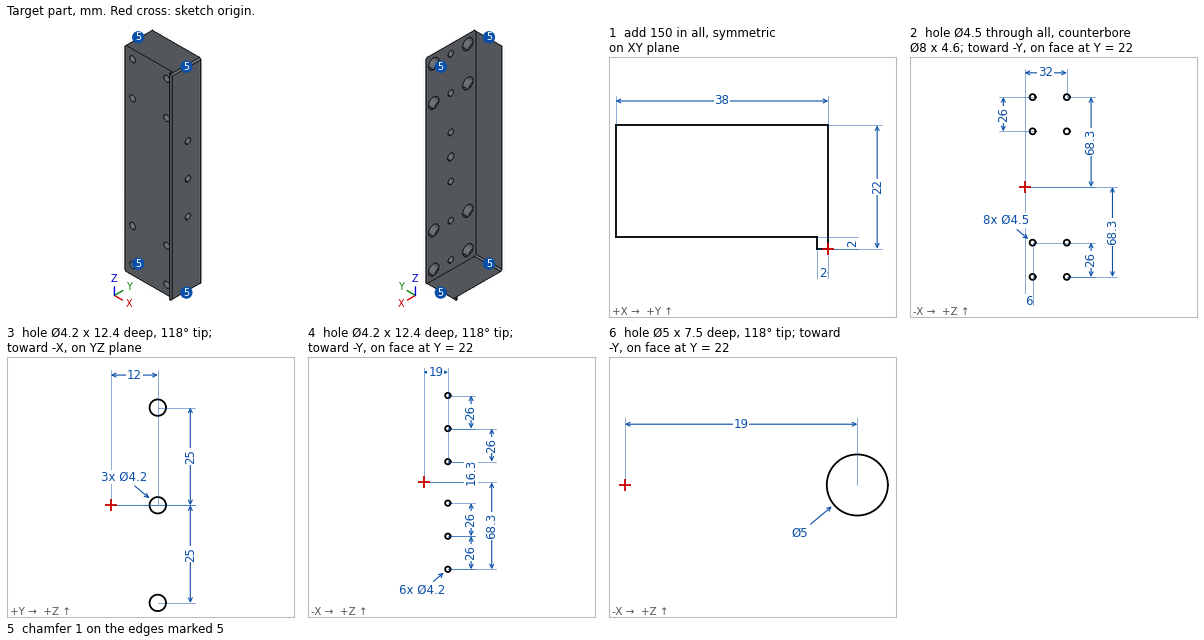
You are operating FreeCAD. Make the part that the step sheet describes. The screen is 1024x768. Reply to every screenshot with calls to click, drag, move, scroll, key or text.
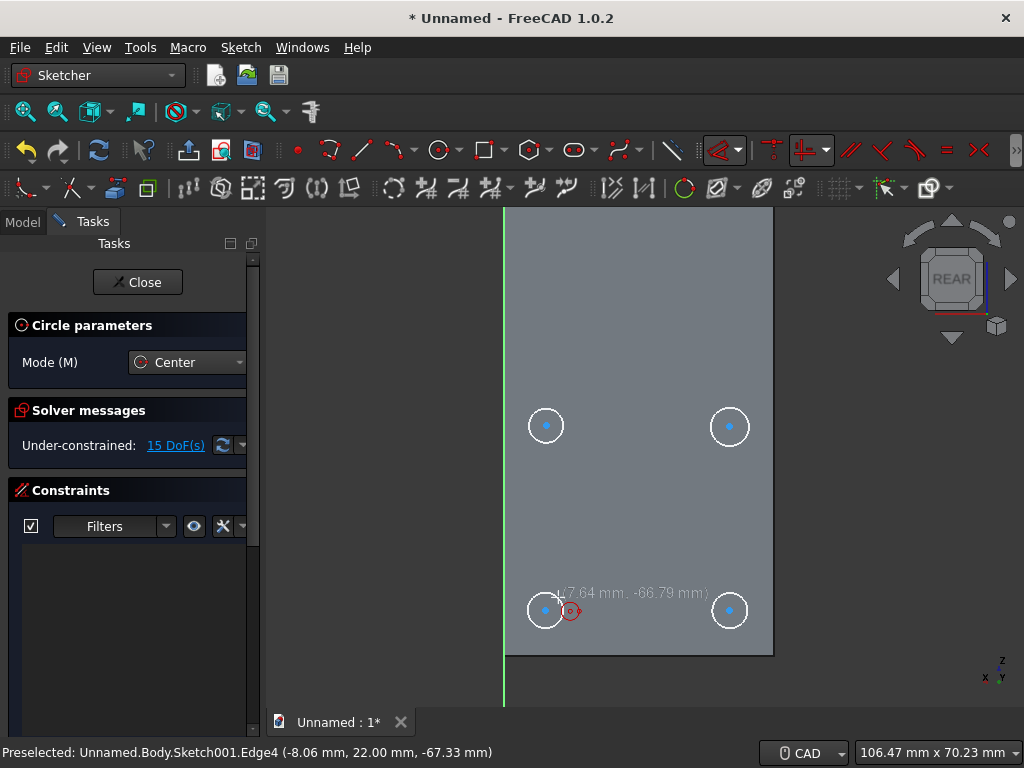
scroll(555, 601, down, 6)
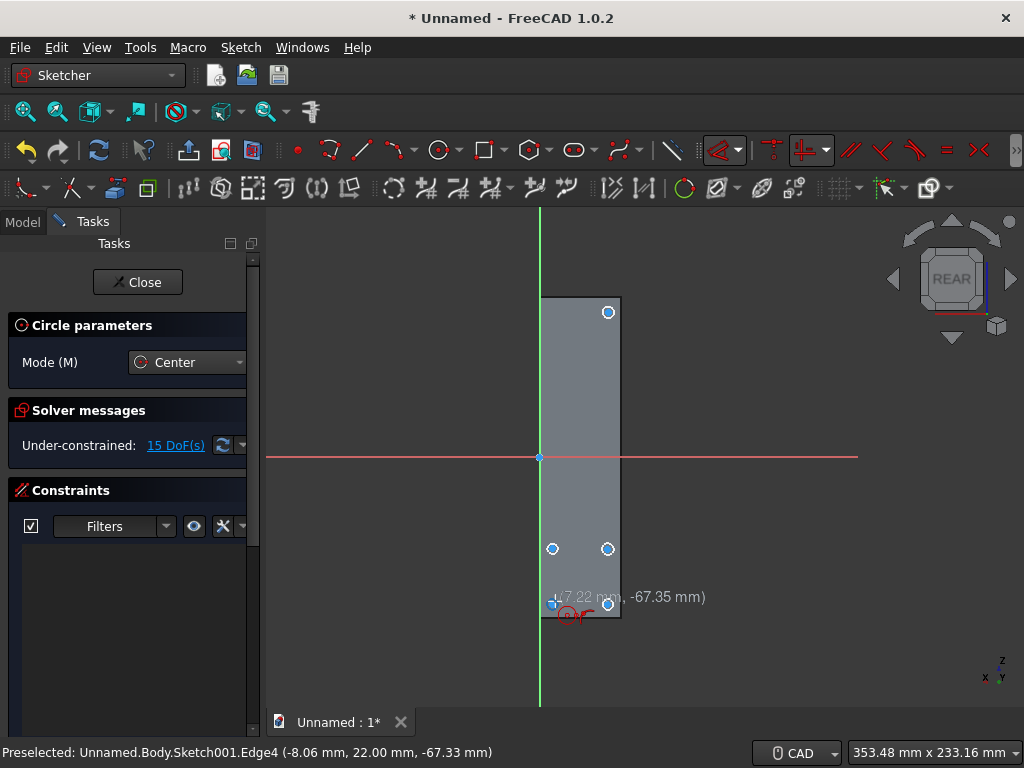
scroll(553, 311, up, 8)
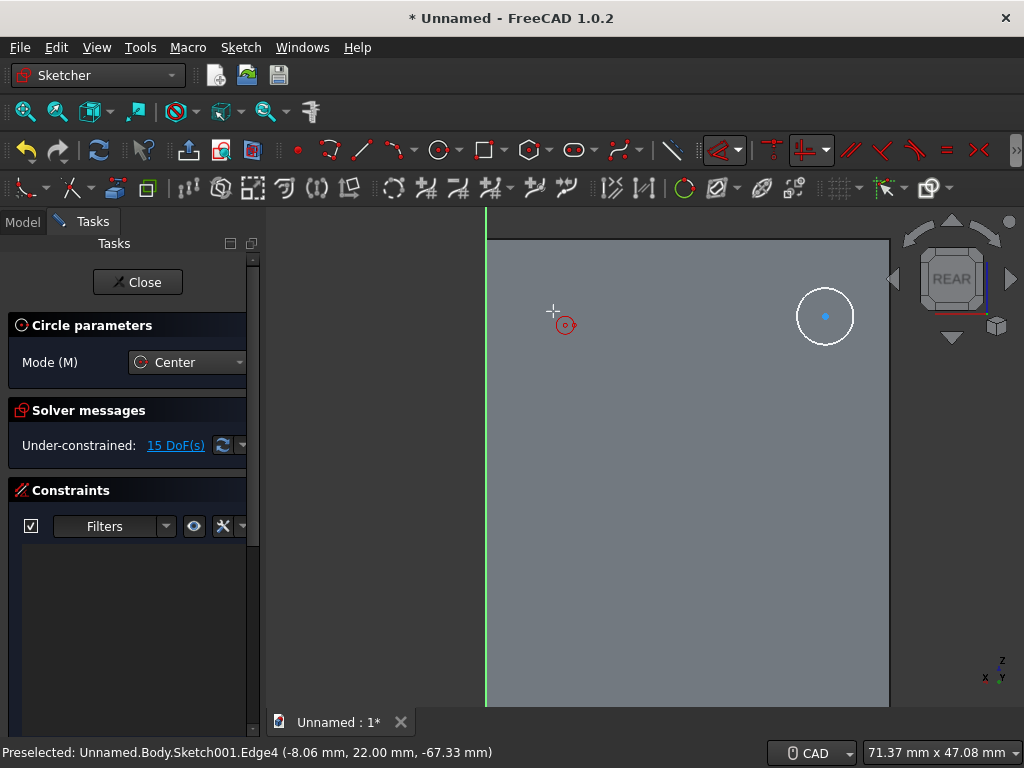
scroll(553, 311, down, 8)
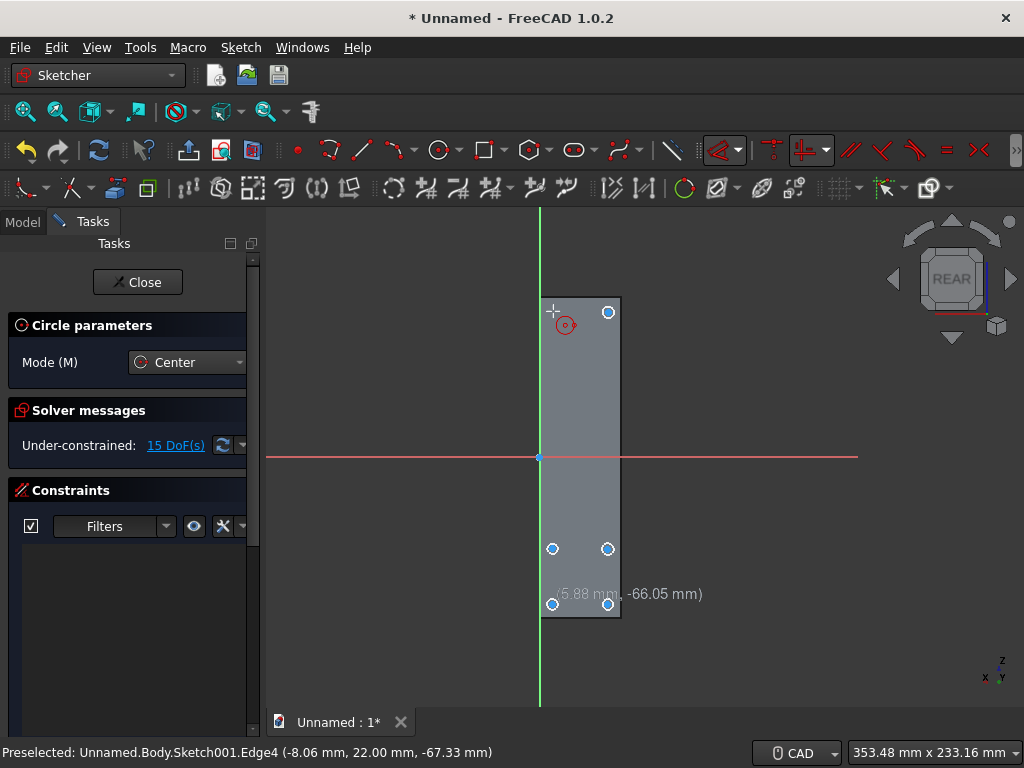
scroll(553, 311, up, 2)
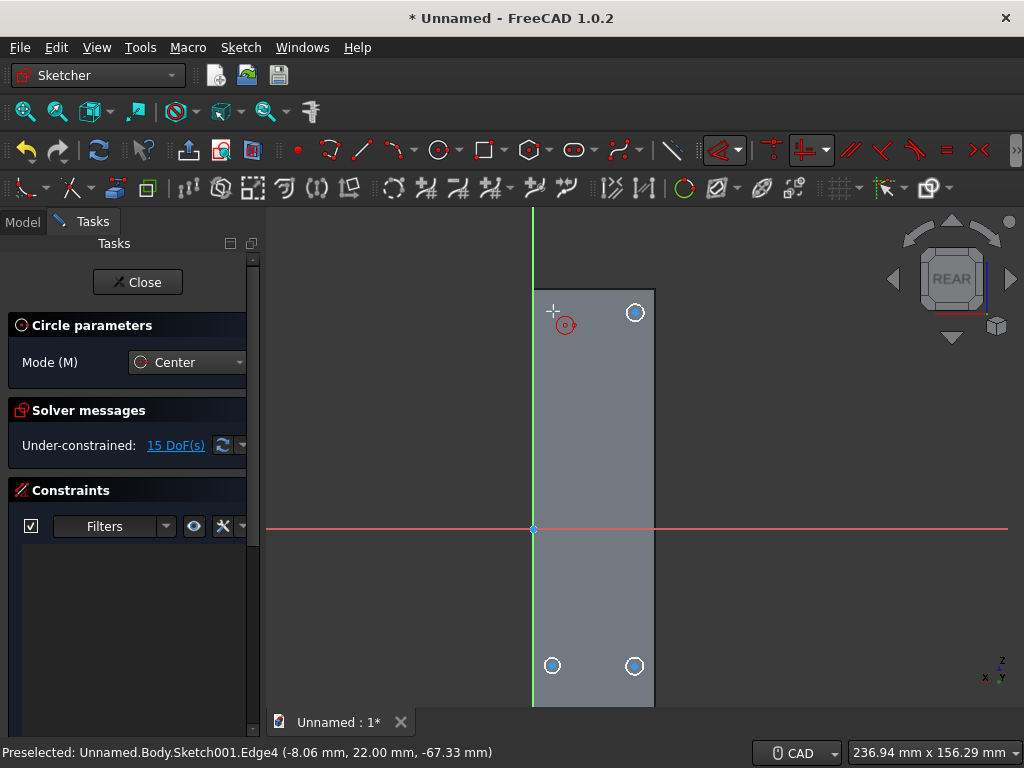
click(552, 311)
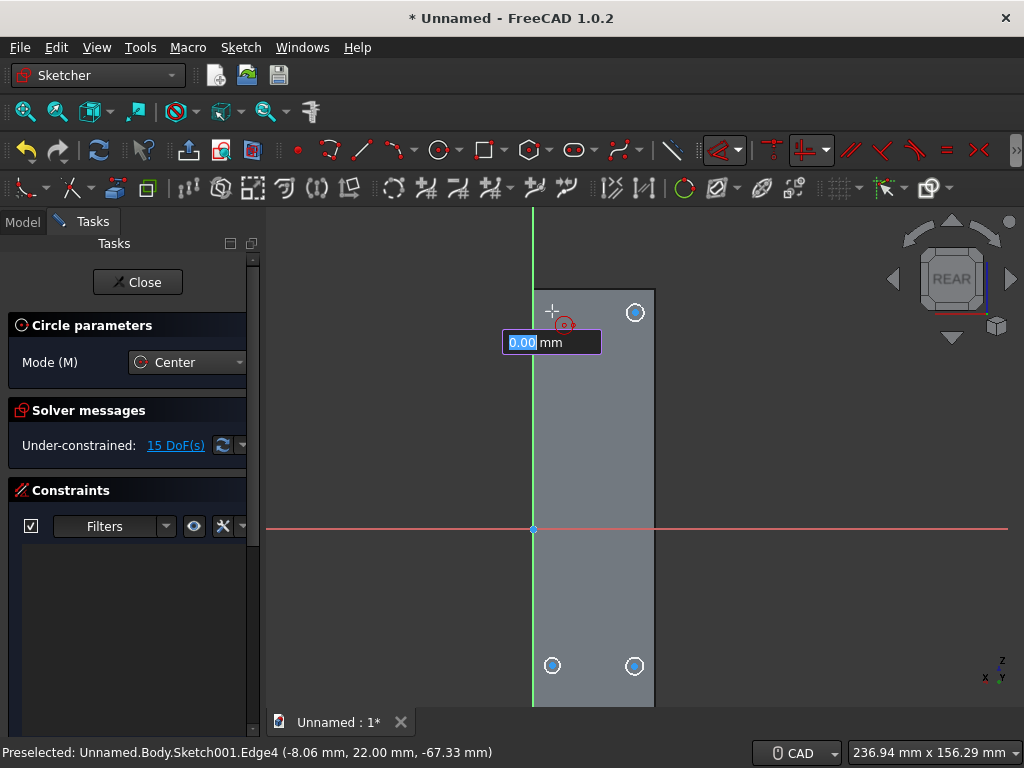
scroll(557, 306, up, 4)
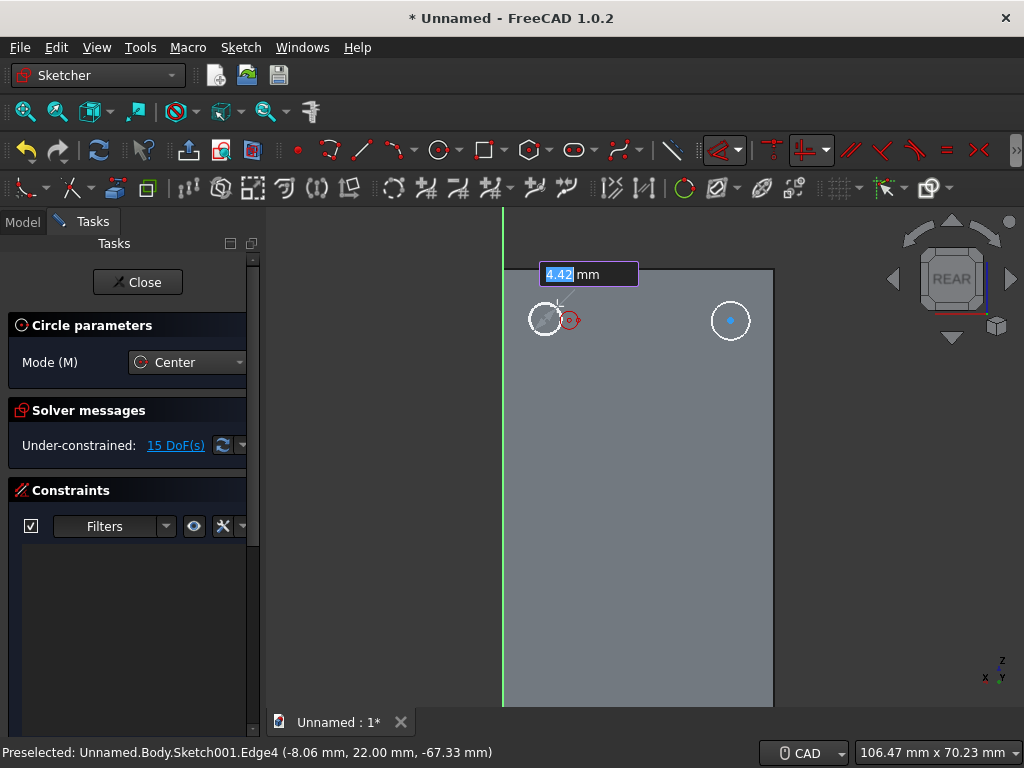
click(557, 305)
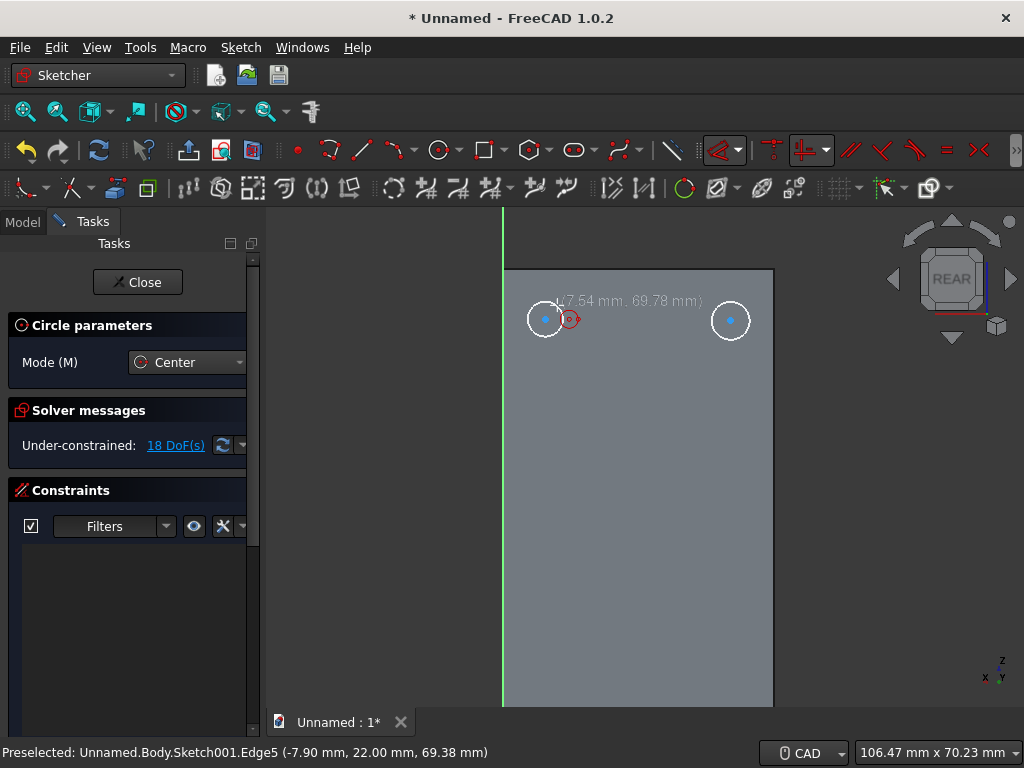
scroll(546, 502, up, 2)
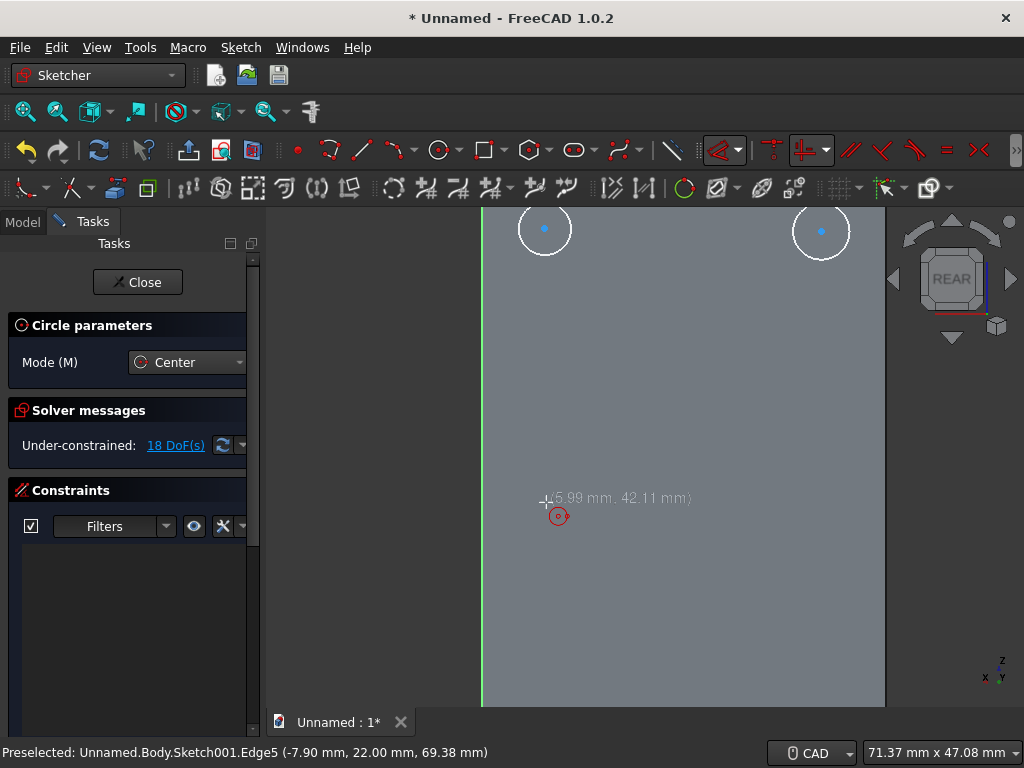
scroll(554, 332, down, 8)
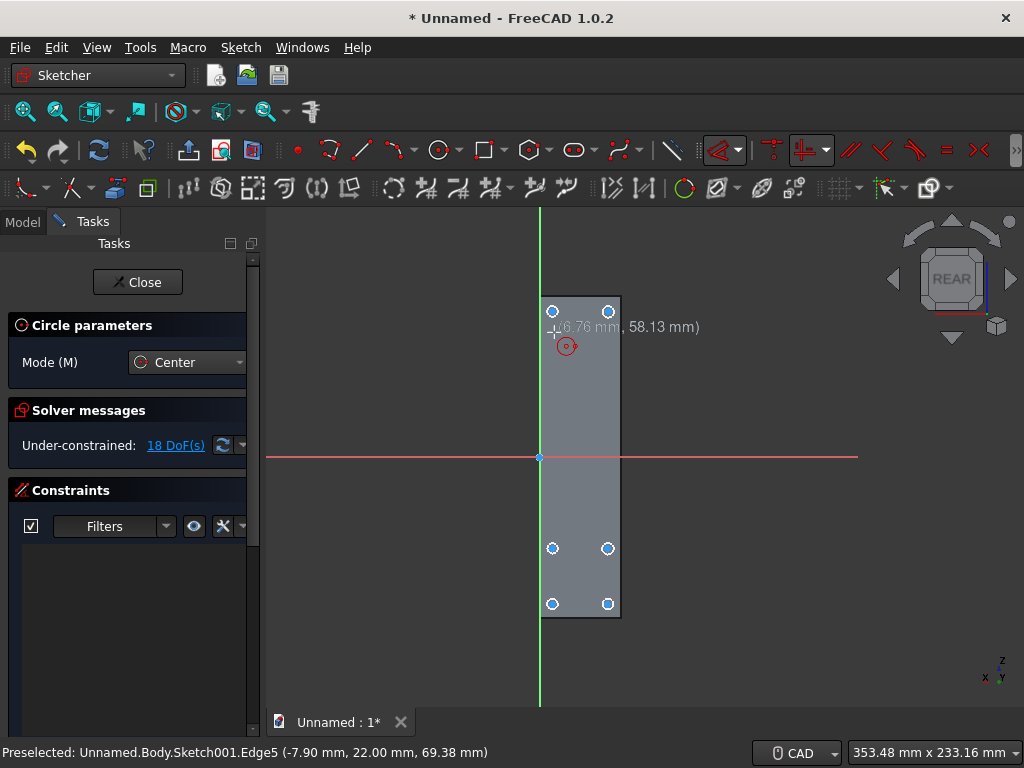
scroll(553, 366, up, 2)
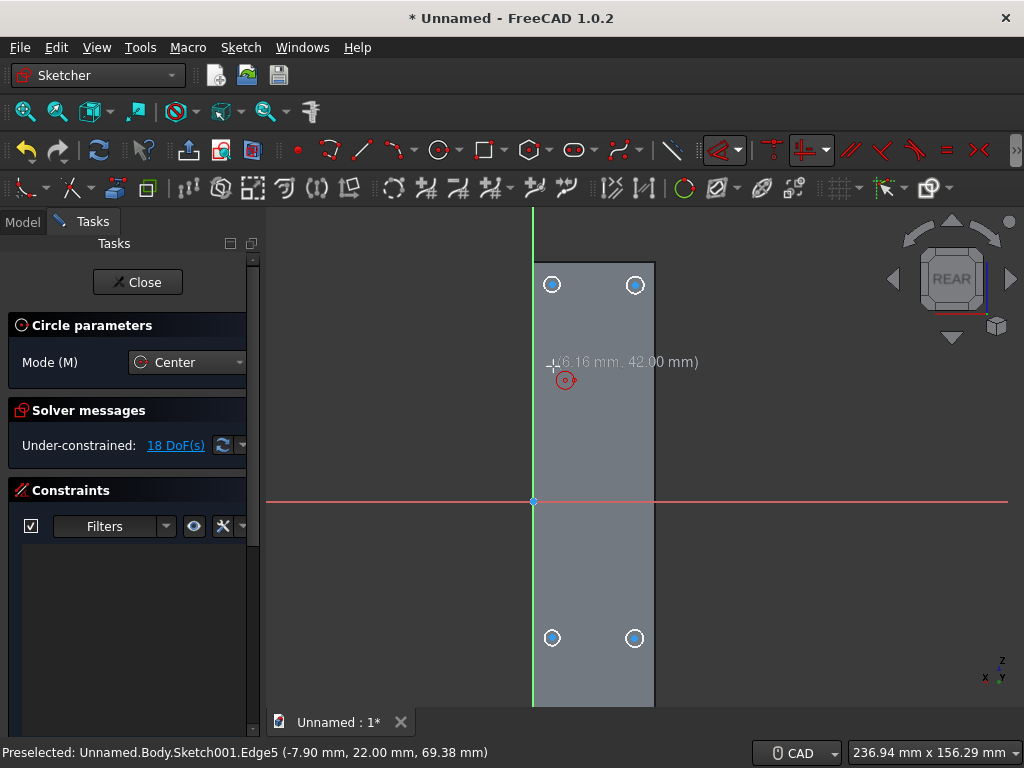
click(552, 366)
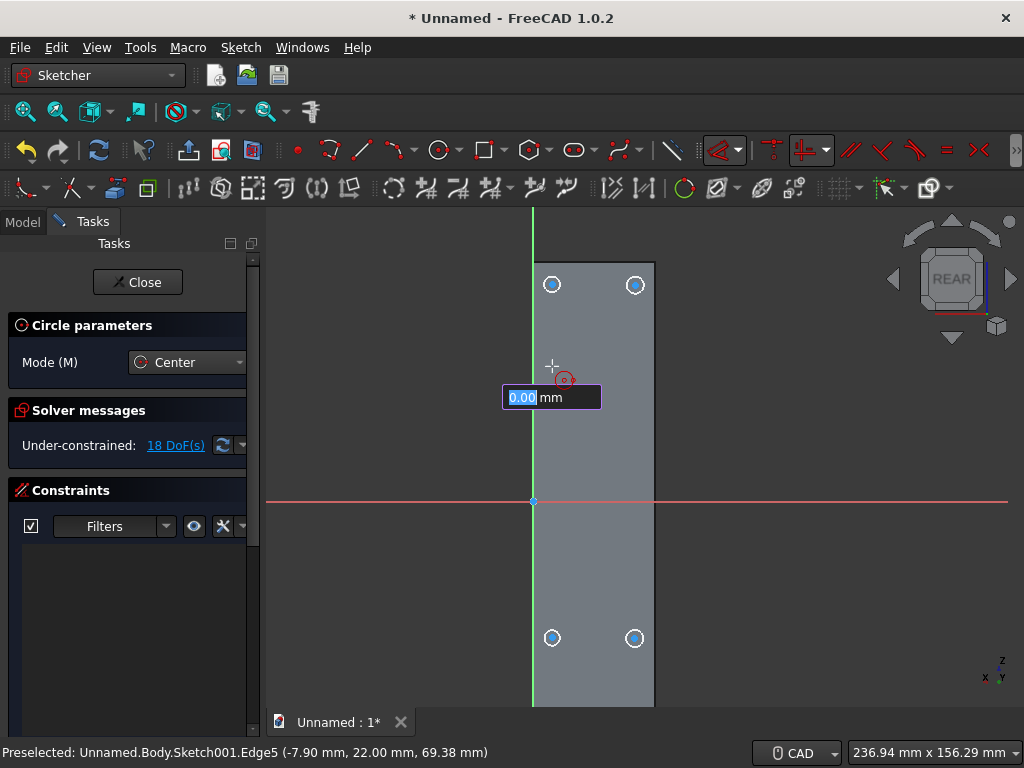
scroll(557, 361, up, 4)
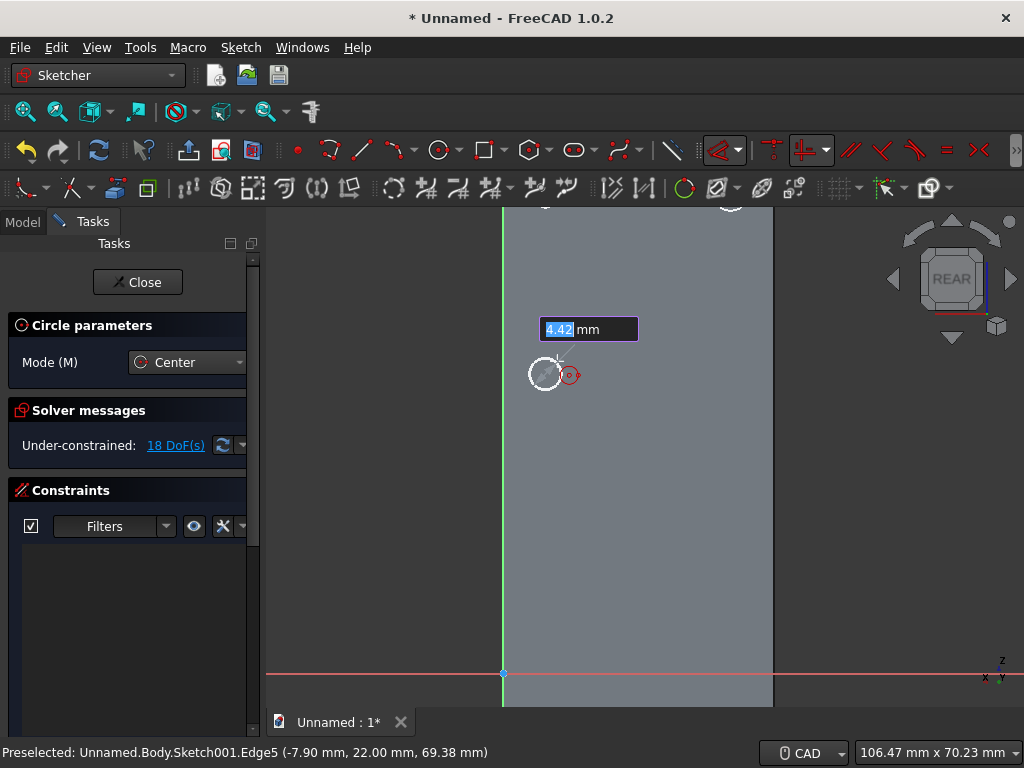
click(557, 361)